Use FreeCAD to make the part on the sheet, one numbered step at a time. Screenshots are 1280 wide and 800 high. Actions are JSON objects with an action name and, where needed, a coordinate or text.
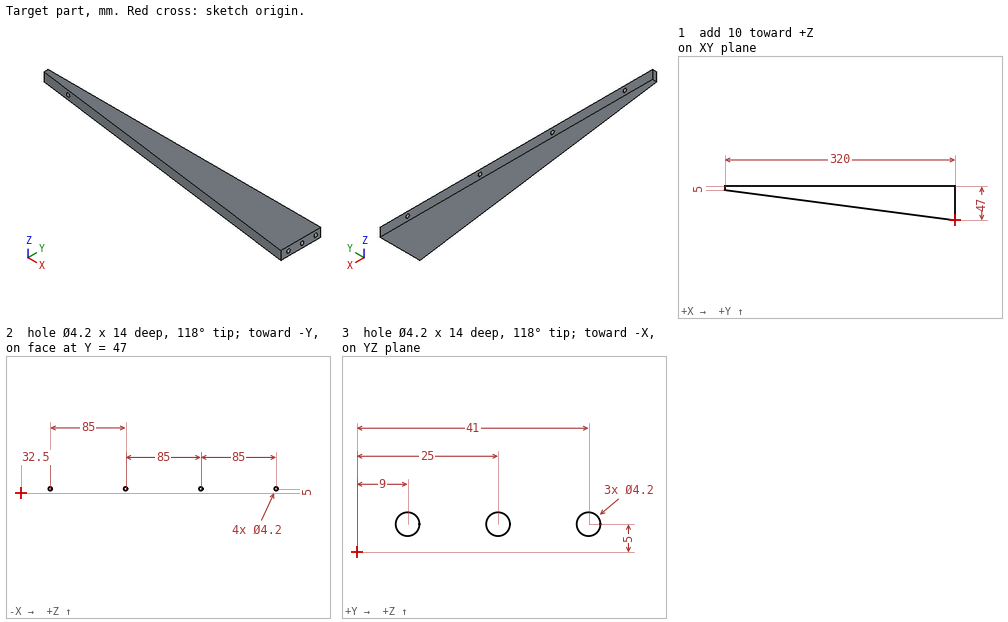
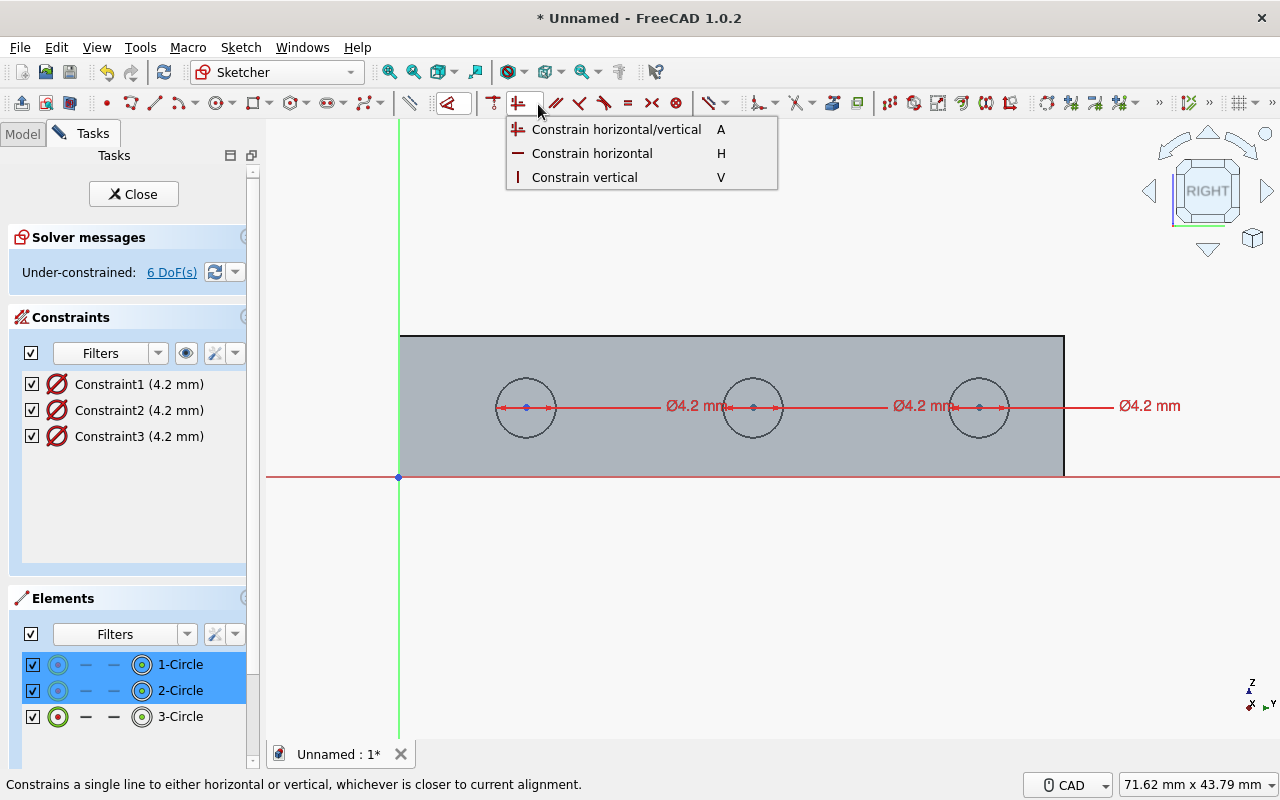
{"action": "left_click", "coordinate": [642, 153]}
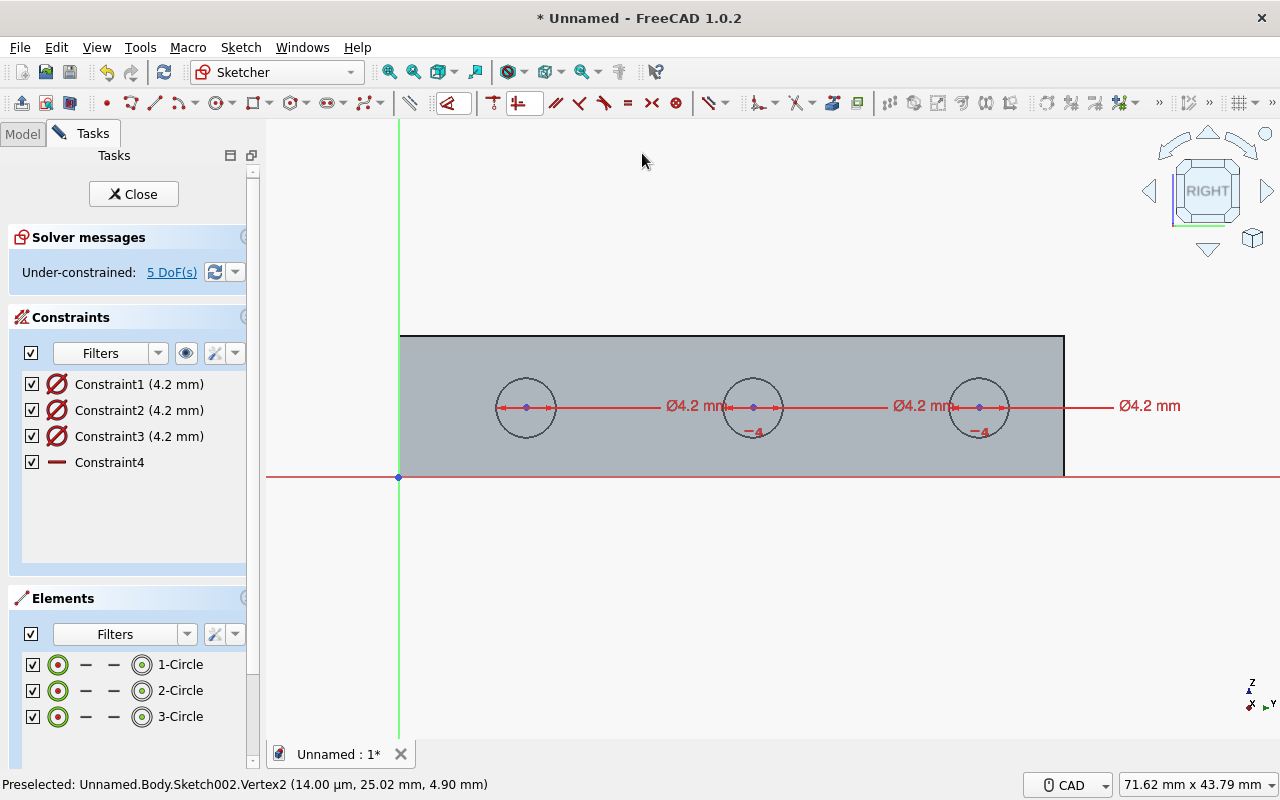
{"action": "left_click", "coordinate": [753, 408]}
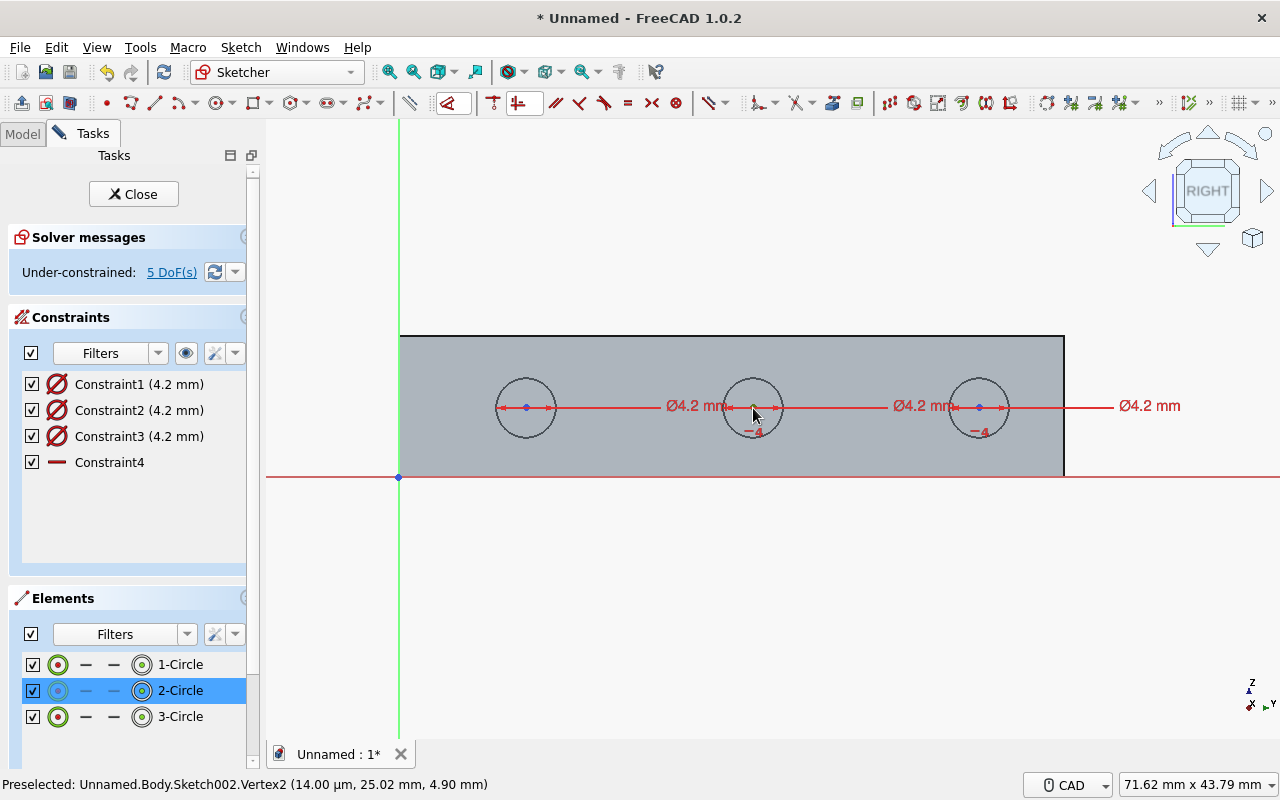
{"action": "left_click", "coordinate": [526, 408]}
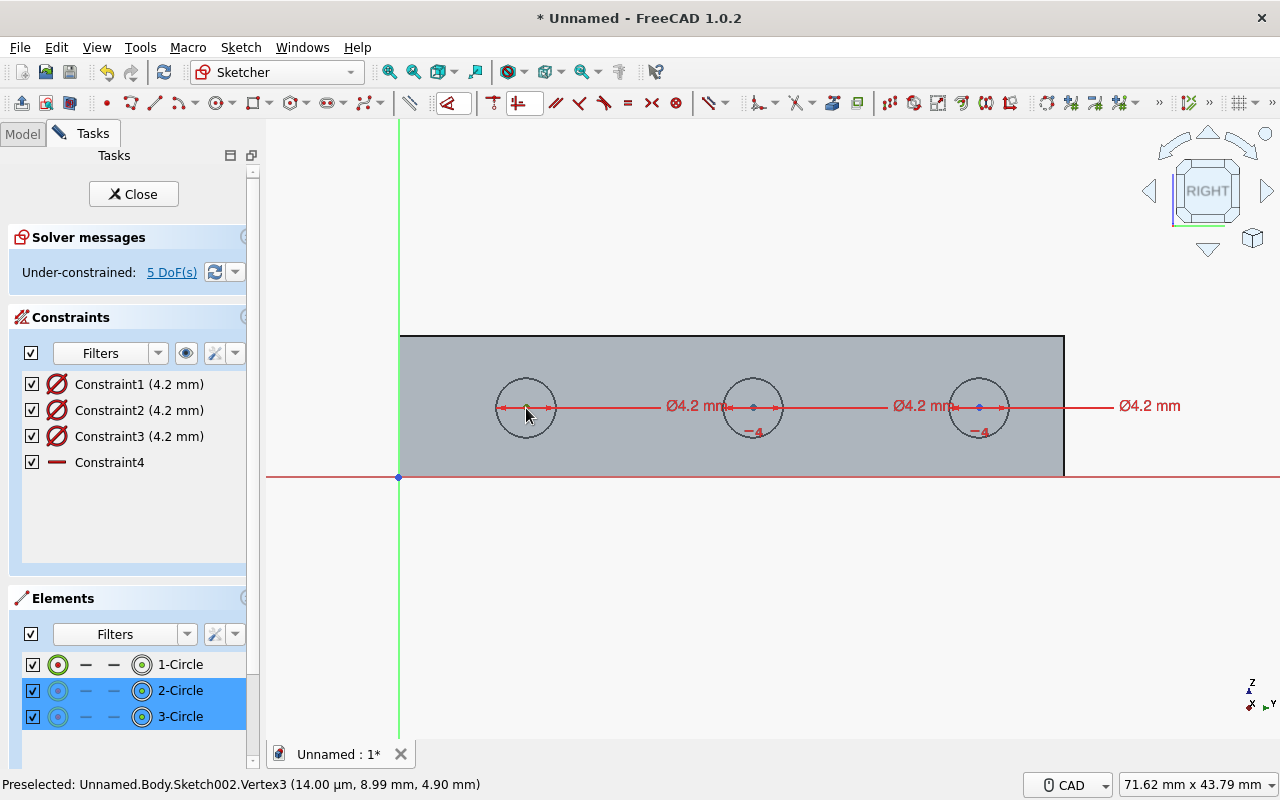
{"action": "left_click", "coordinate": [538, 104]}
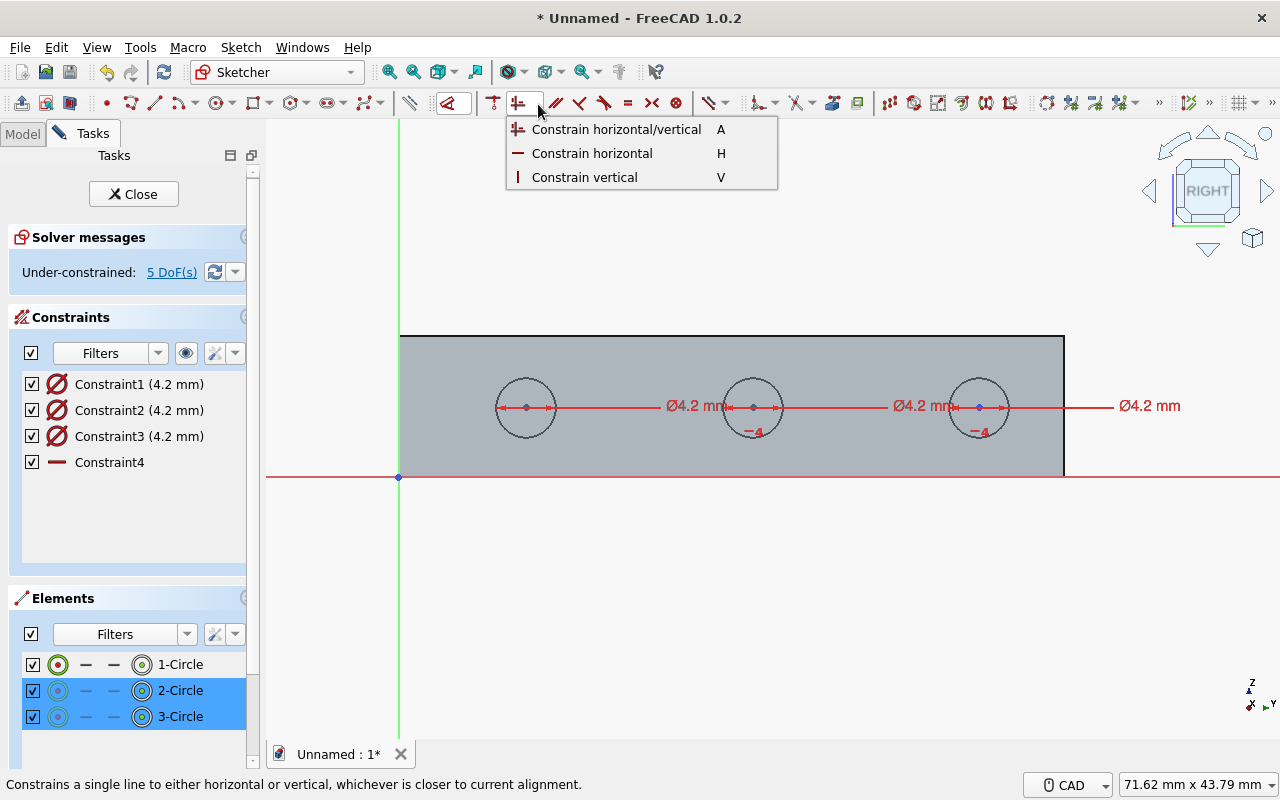
{"action": "left_click", "coordinate": [642, 153]}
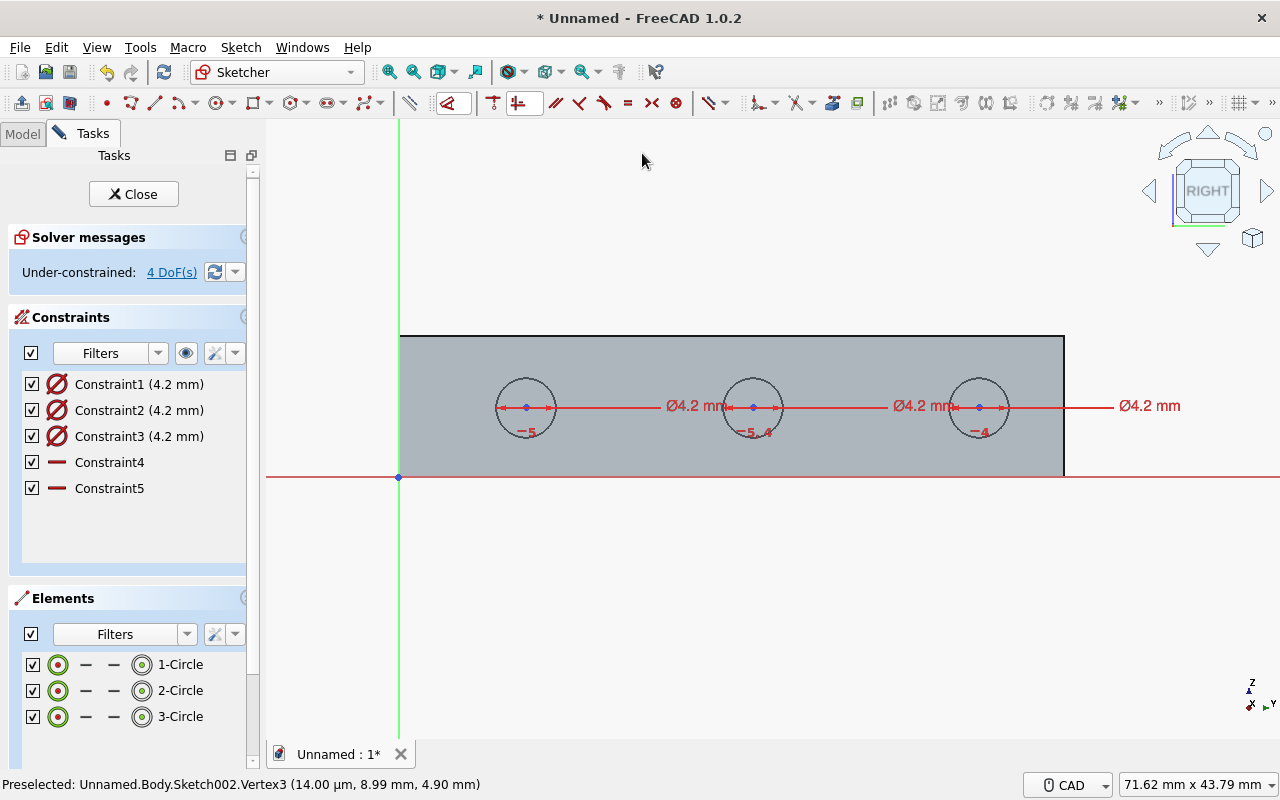
{"action": "left_click", "coordinate": [448, 104]}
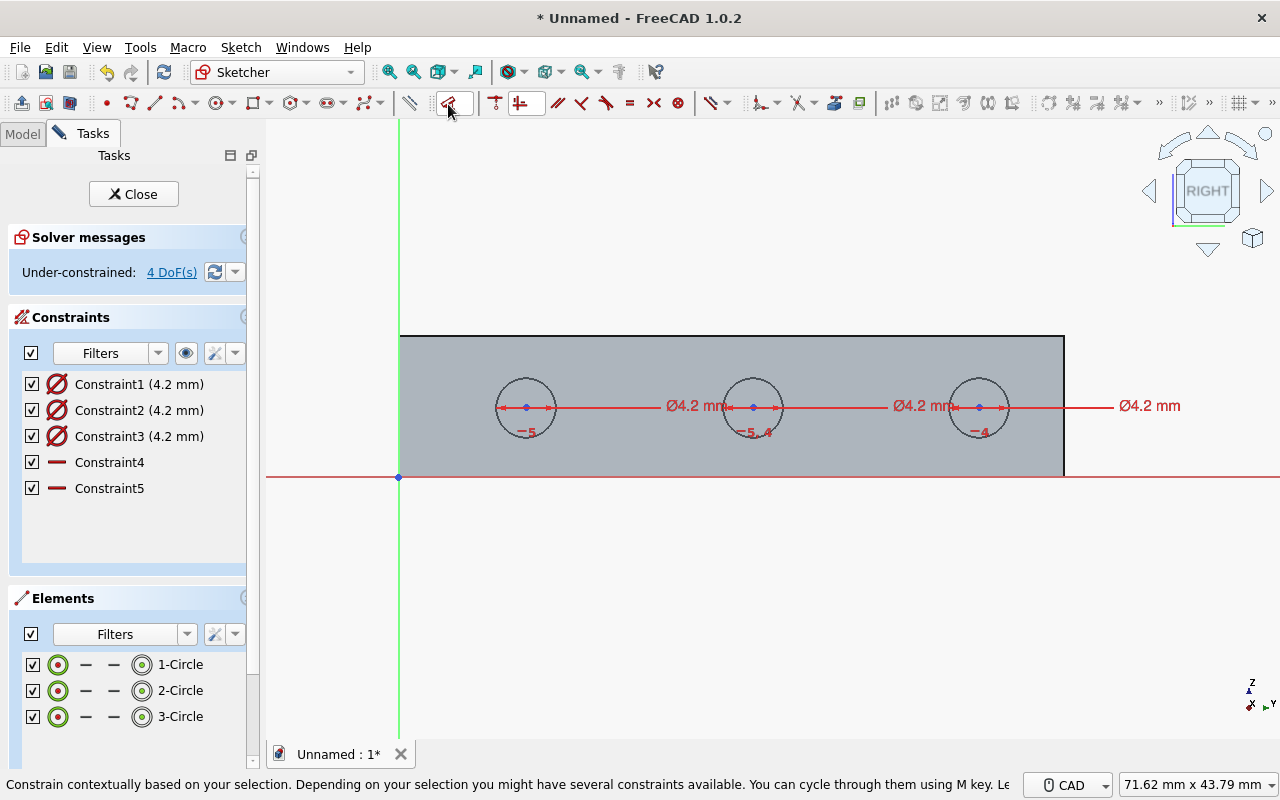
{"action": "left_click", "coordinate": [979, 408]}
{"action": "left_click", "coordinate": [365, 443]}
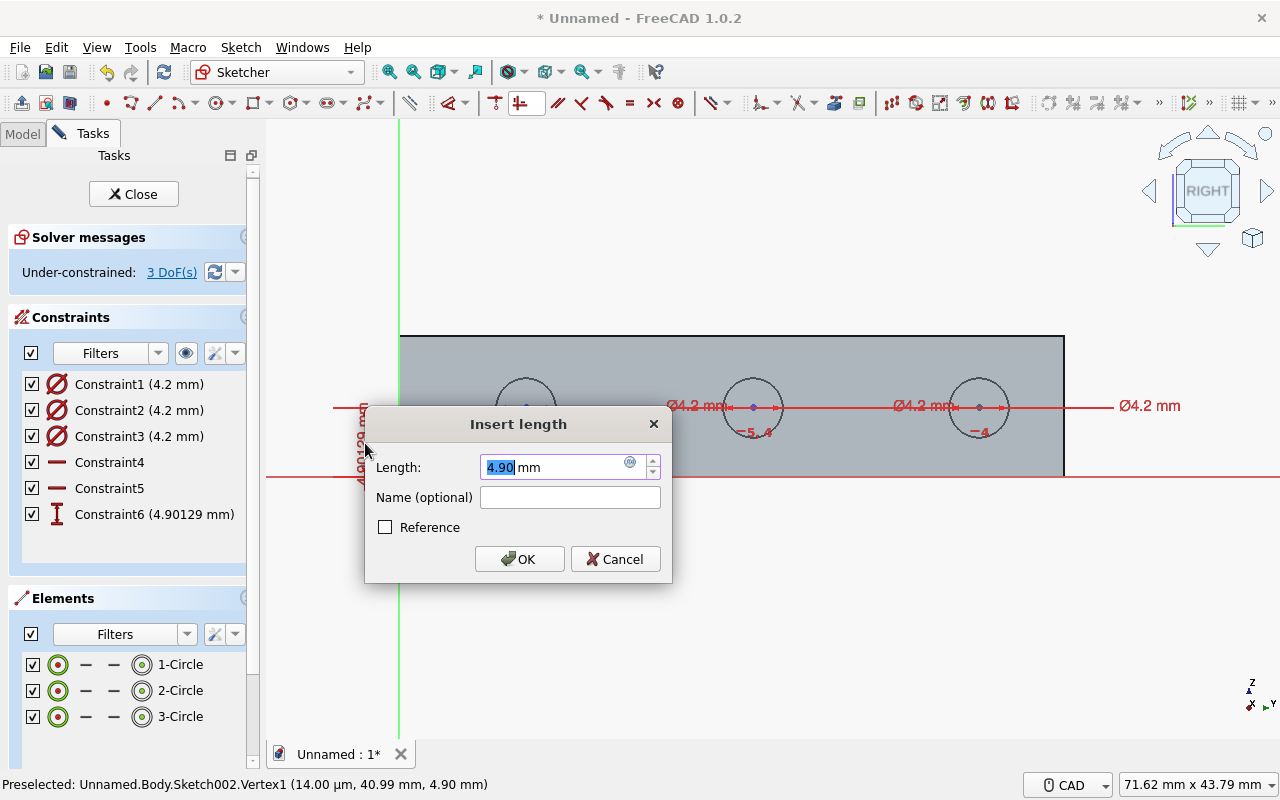
{"action": "type", "text": "5"}
{"action": "key", "text": "Return"}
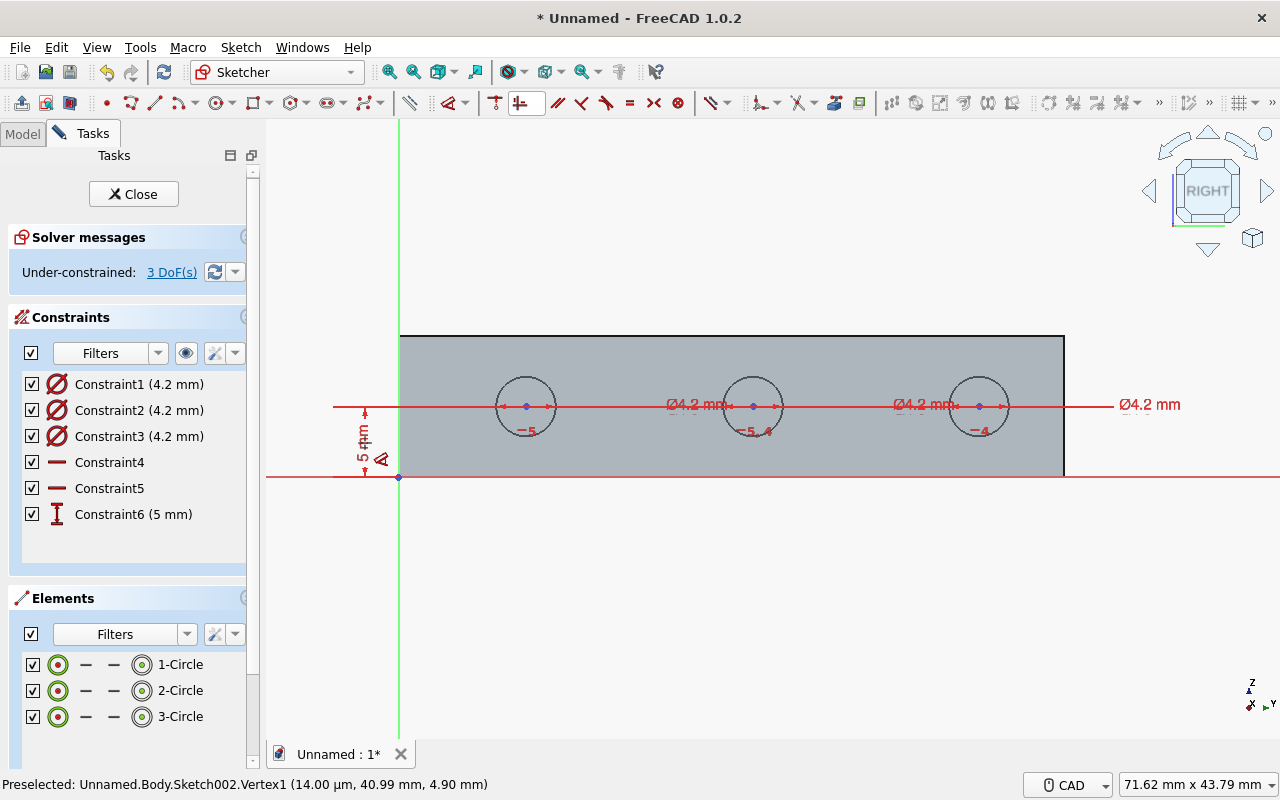
{"action": "left_click", "coordinate": [526, 407]}
{"action": "left_click", "coordinate": [462, 511]}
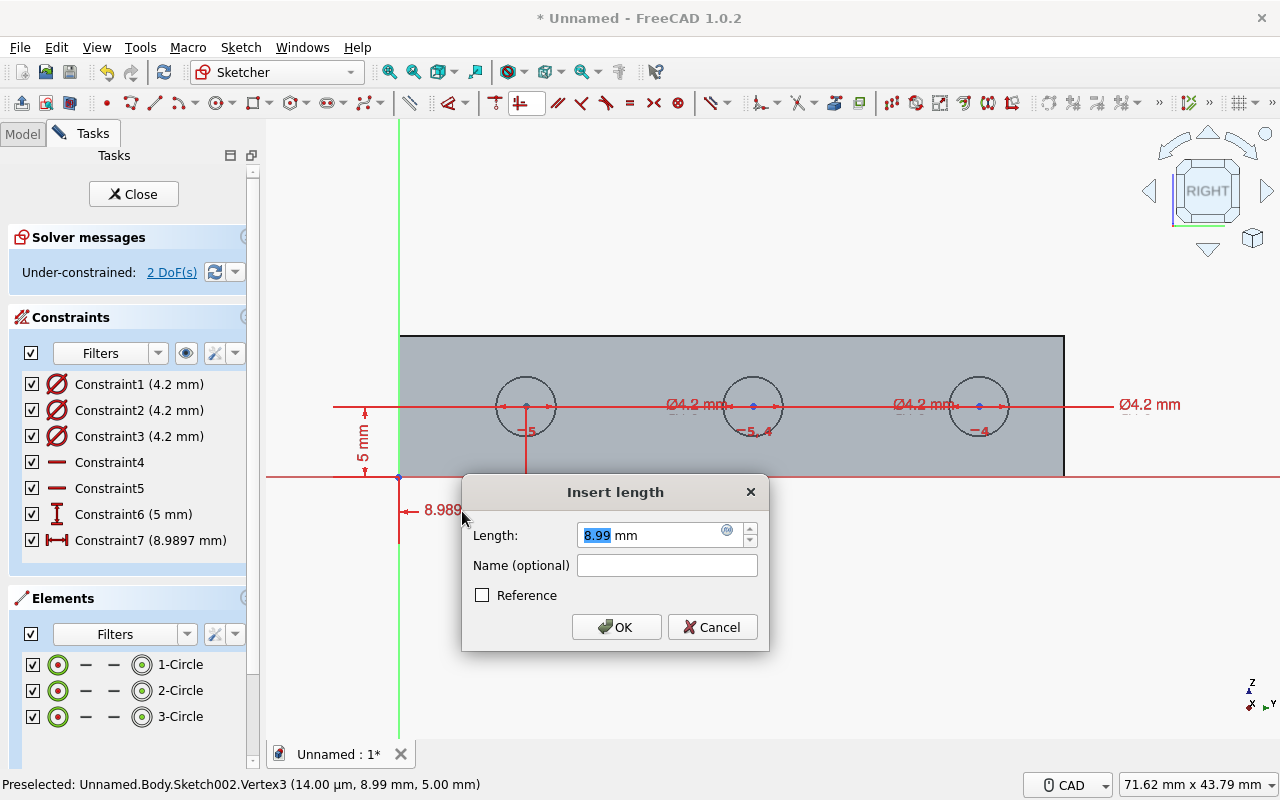
{"action": "type", "text": "9"}
{"action": "key", "text": "Return"}